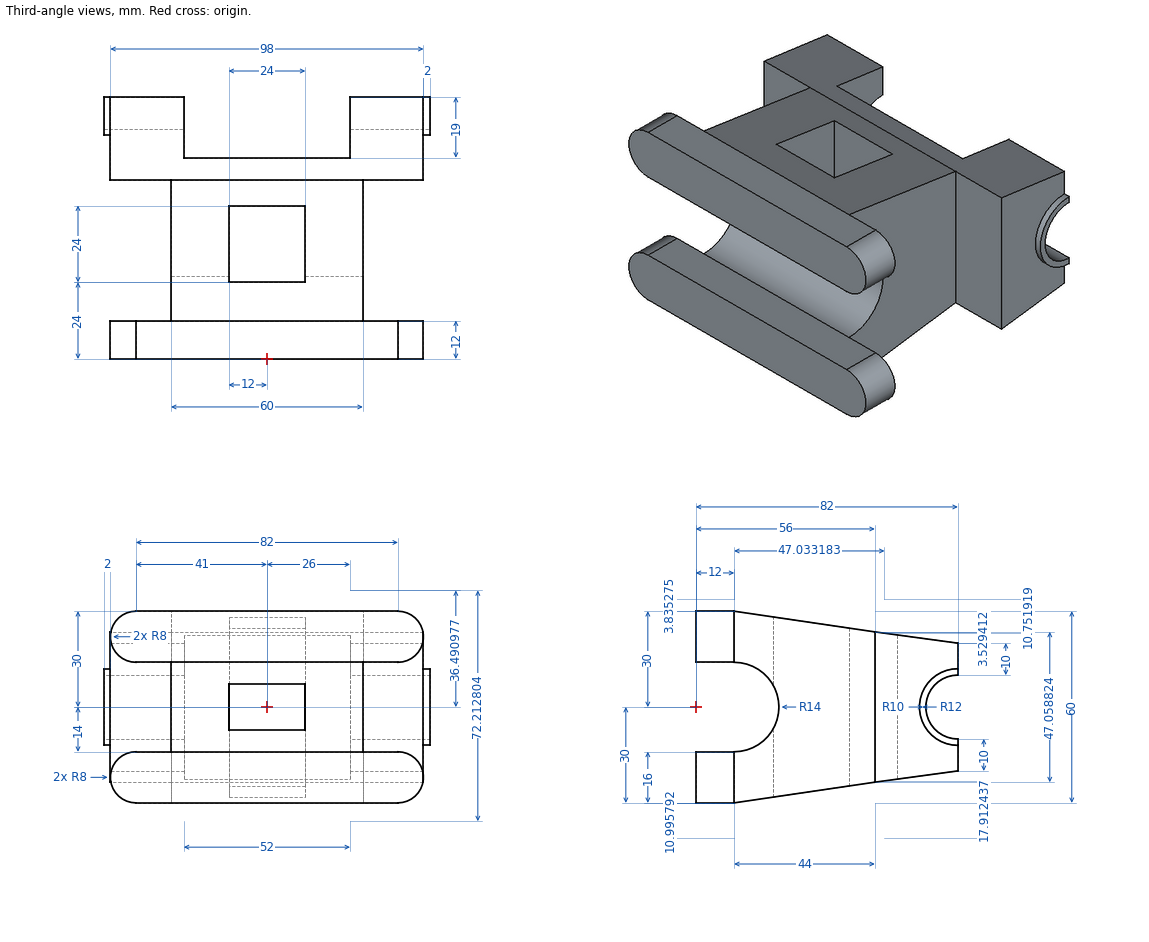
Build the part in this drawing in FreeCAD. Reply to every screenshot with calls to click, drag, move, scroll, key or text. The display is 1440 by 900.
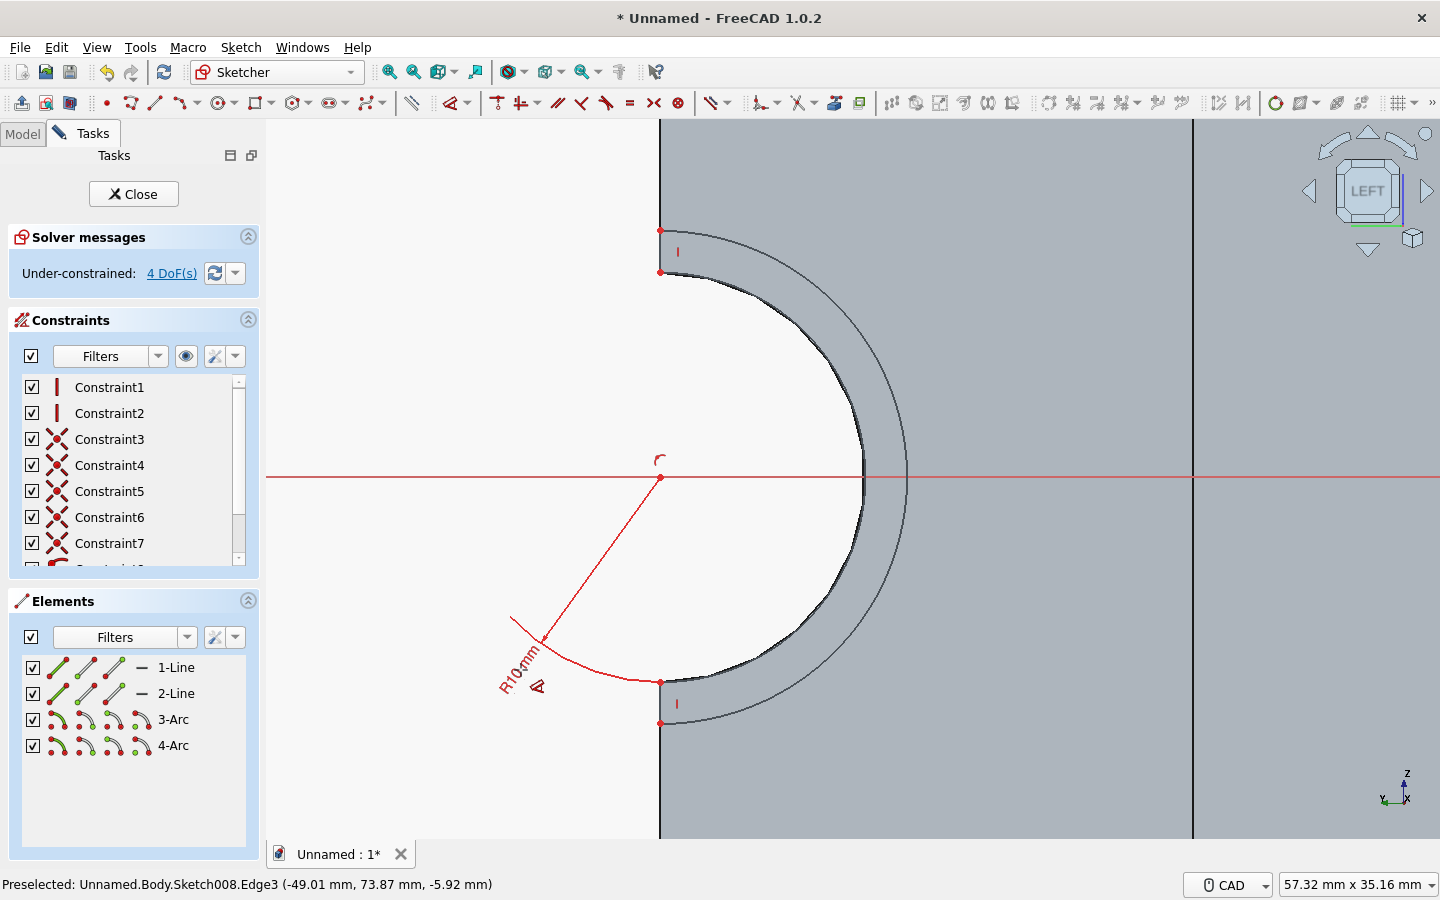
click(860, 623)
click(886, 642)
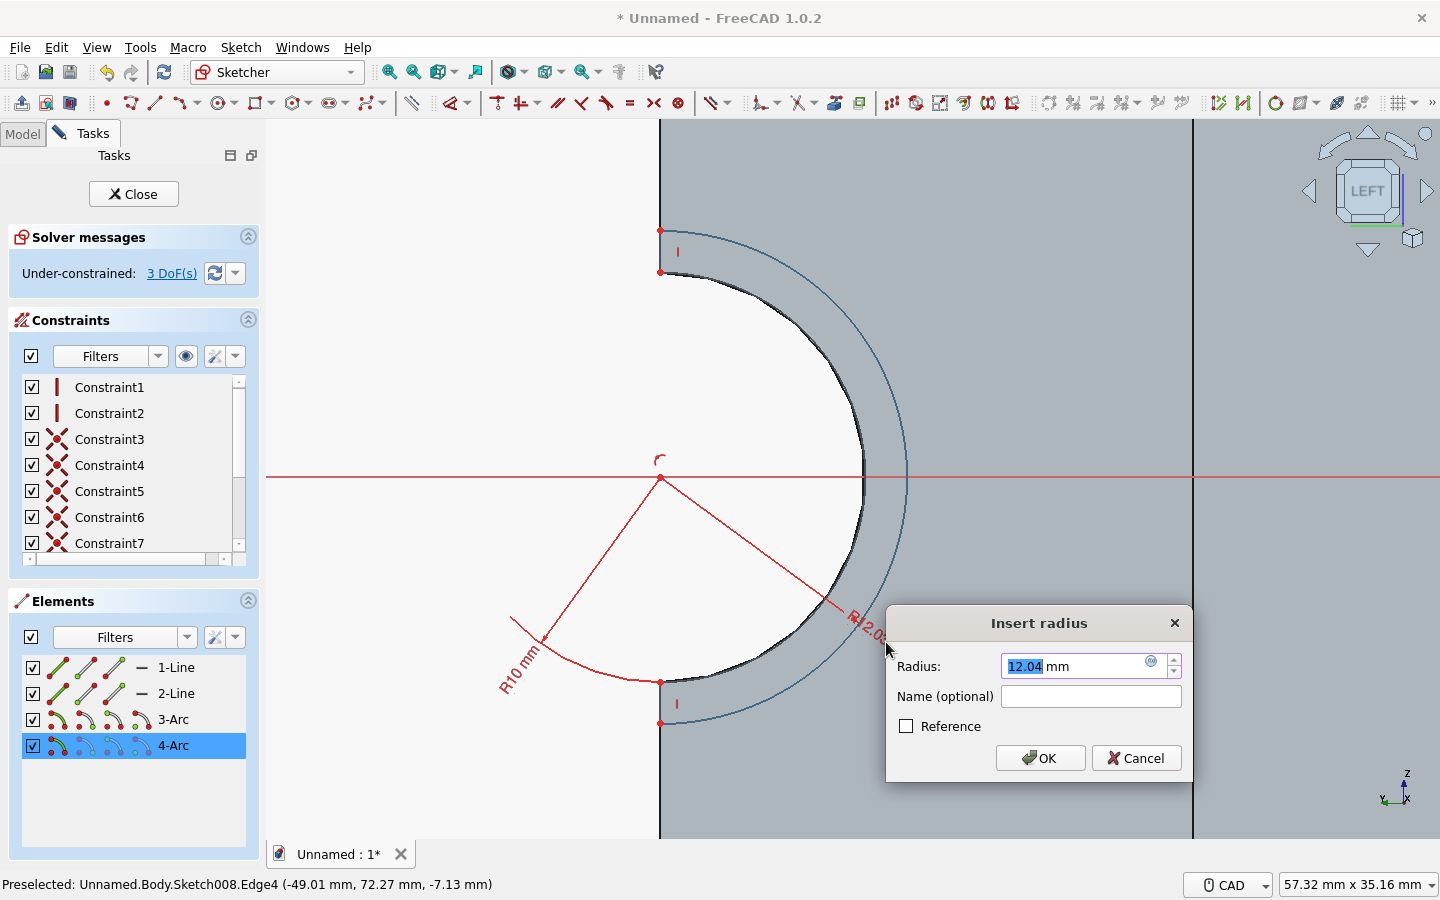
text(12)
key(Return)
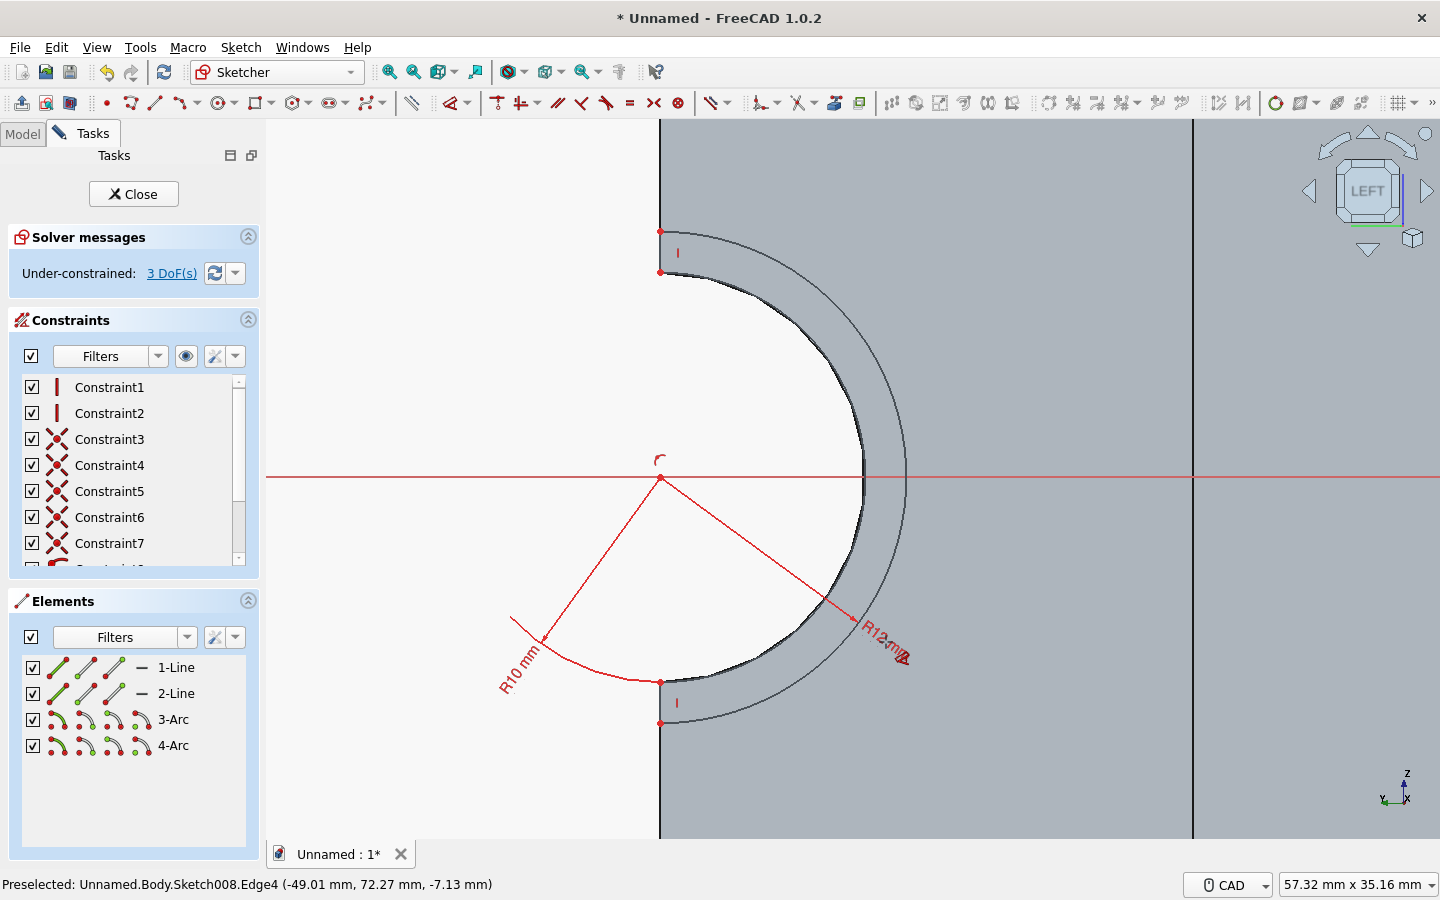
click(660, 232)
click(968, 198)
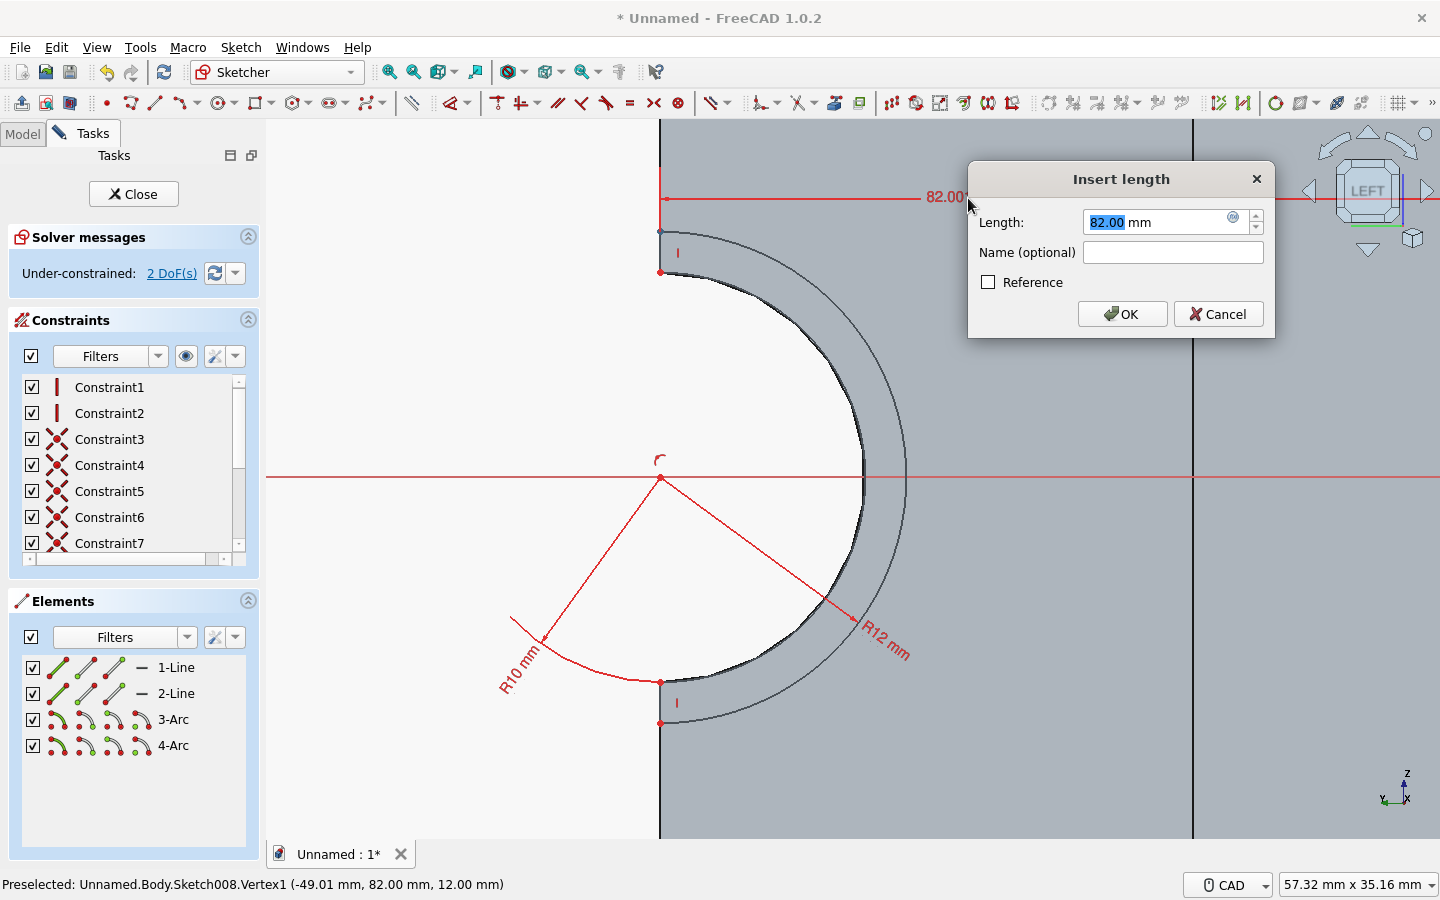
text(82)
key(Return)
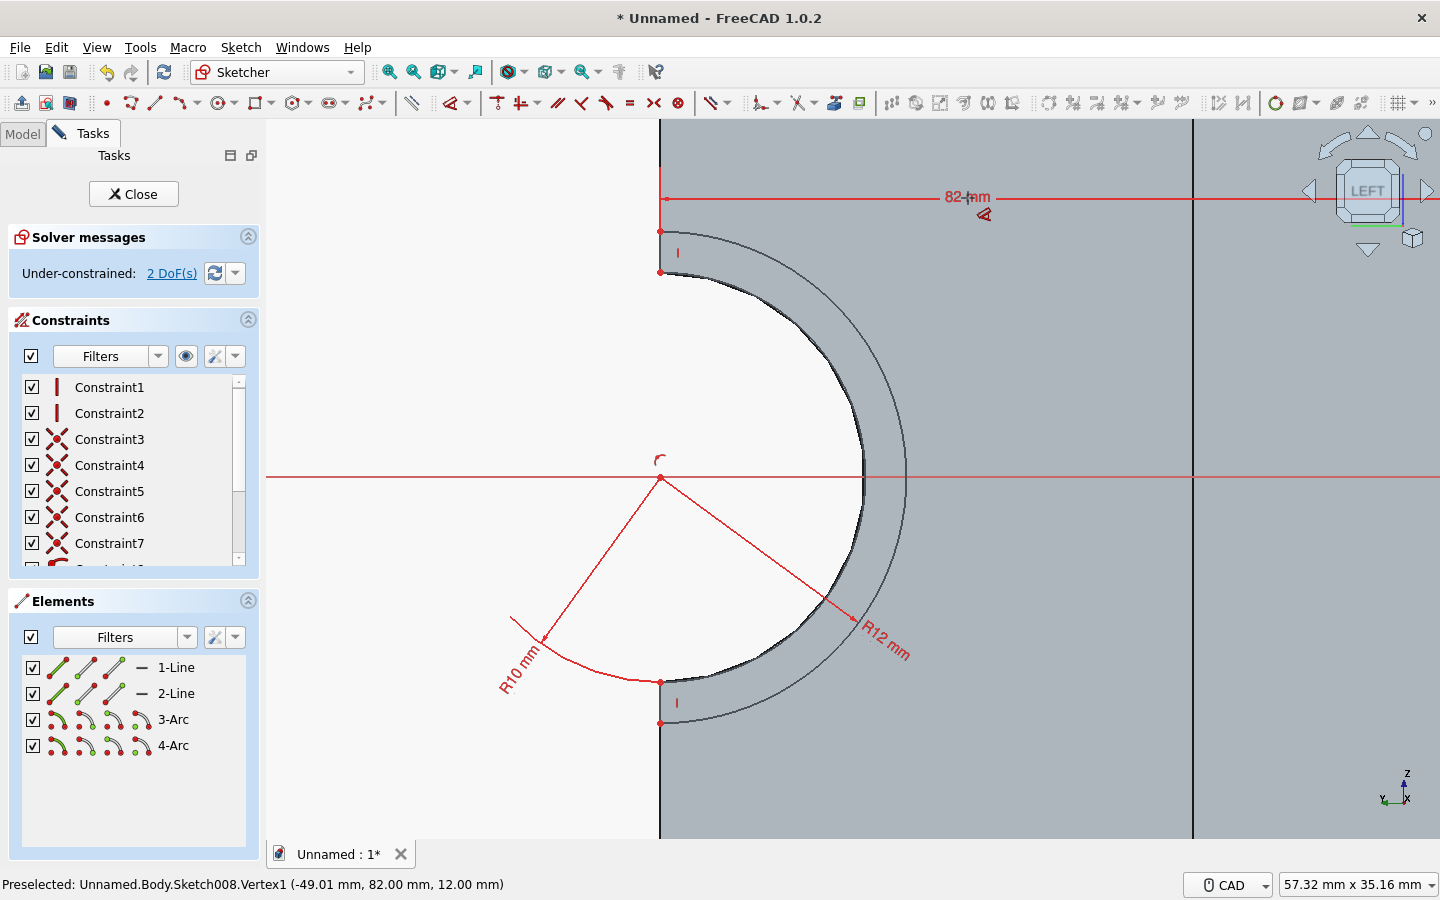
click(660, 682)
click(967, 716)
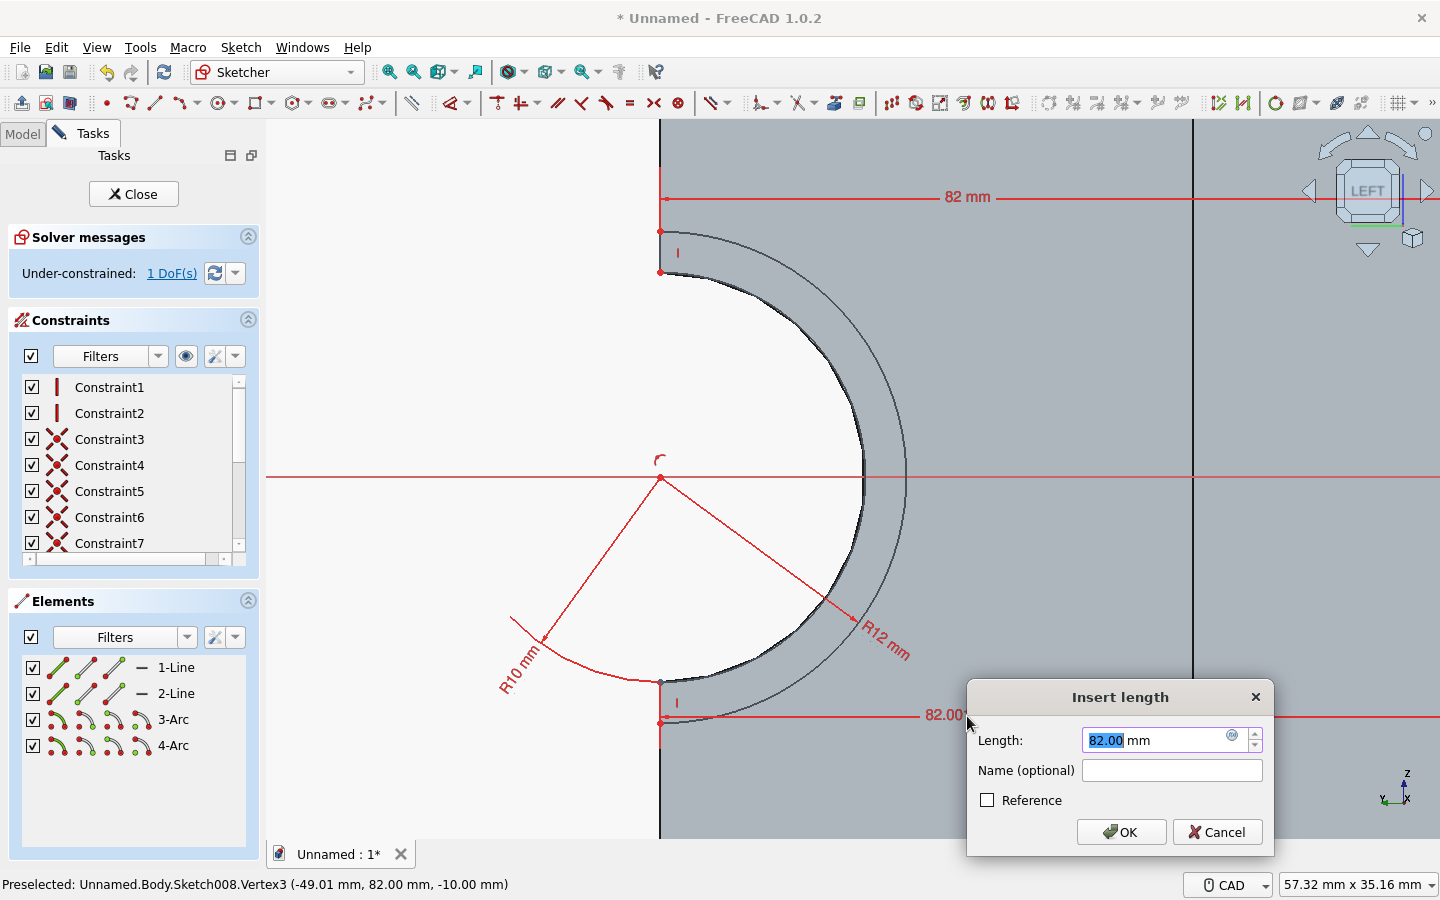
text(82)
key(Return)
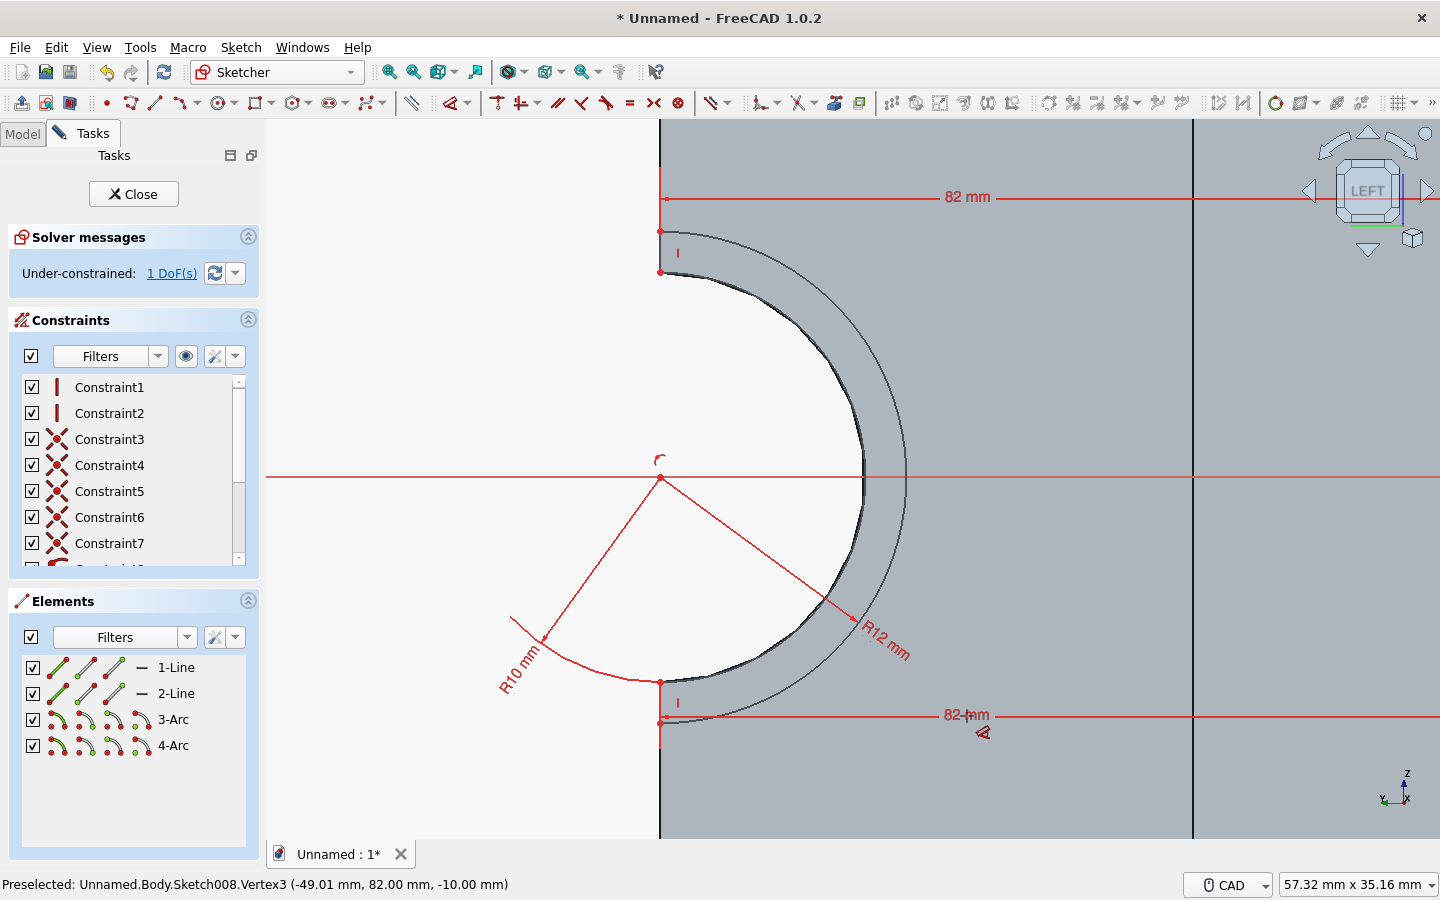
click(661, 477)
click(968, 511)